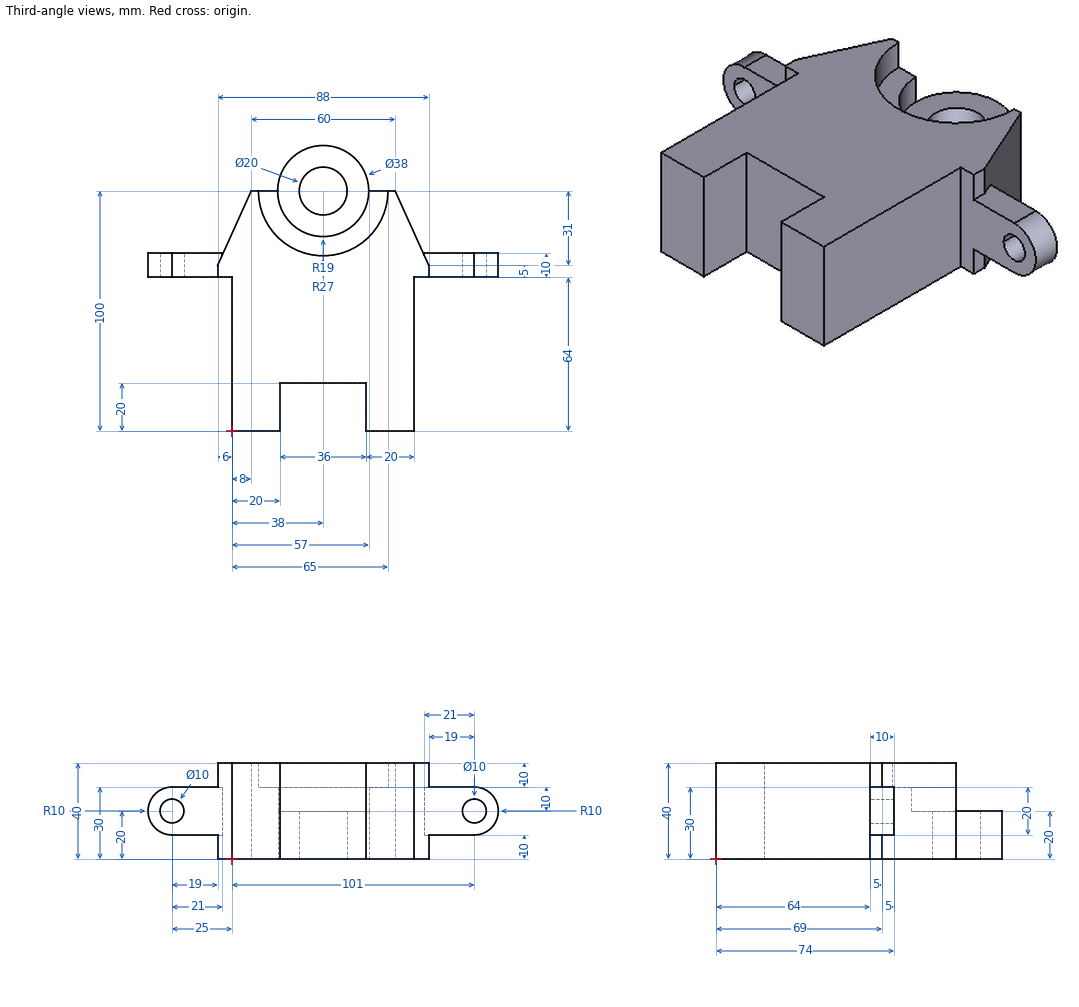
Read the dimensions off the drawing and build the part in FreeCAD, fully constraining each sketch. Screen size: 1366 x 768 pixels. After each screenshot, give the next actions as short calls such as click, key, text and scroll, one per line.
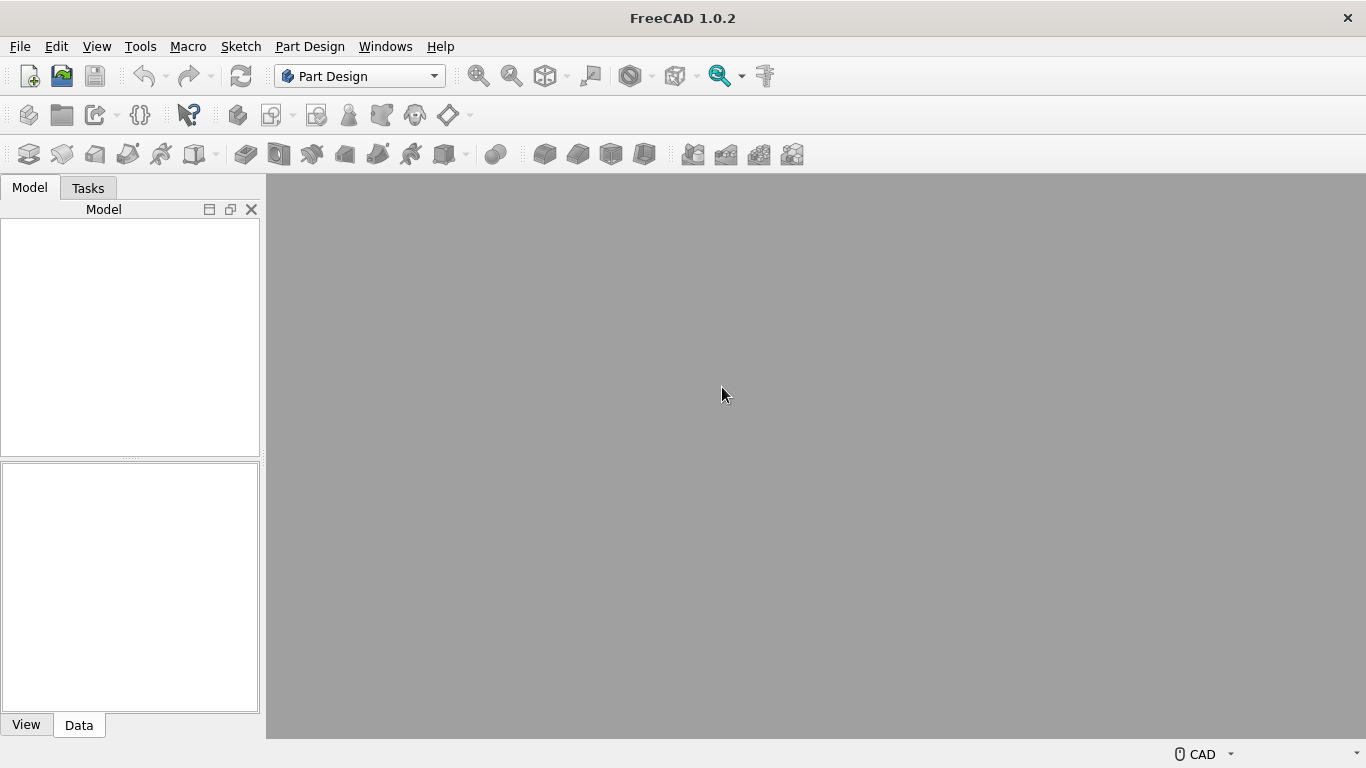
click(29, 76)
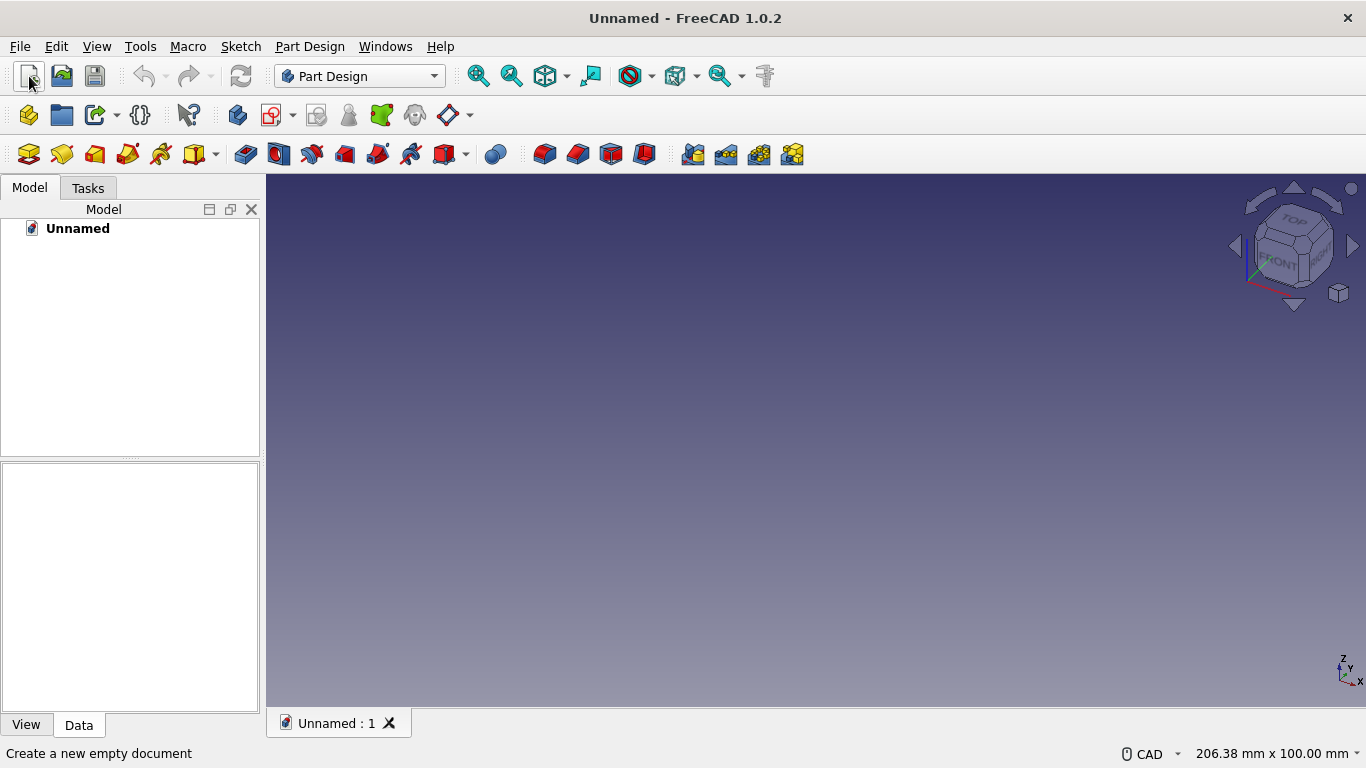
click(270, 116)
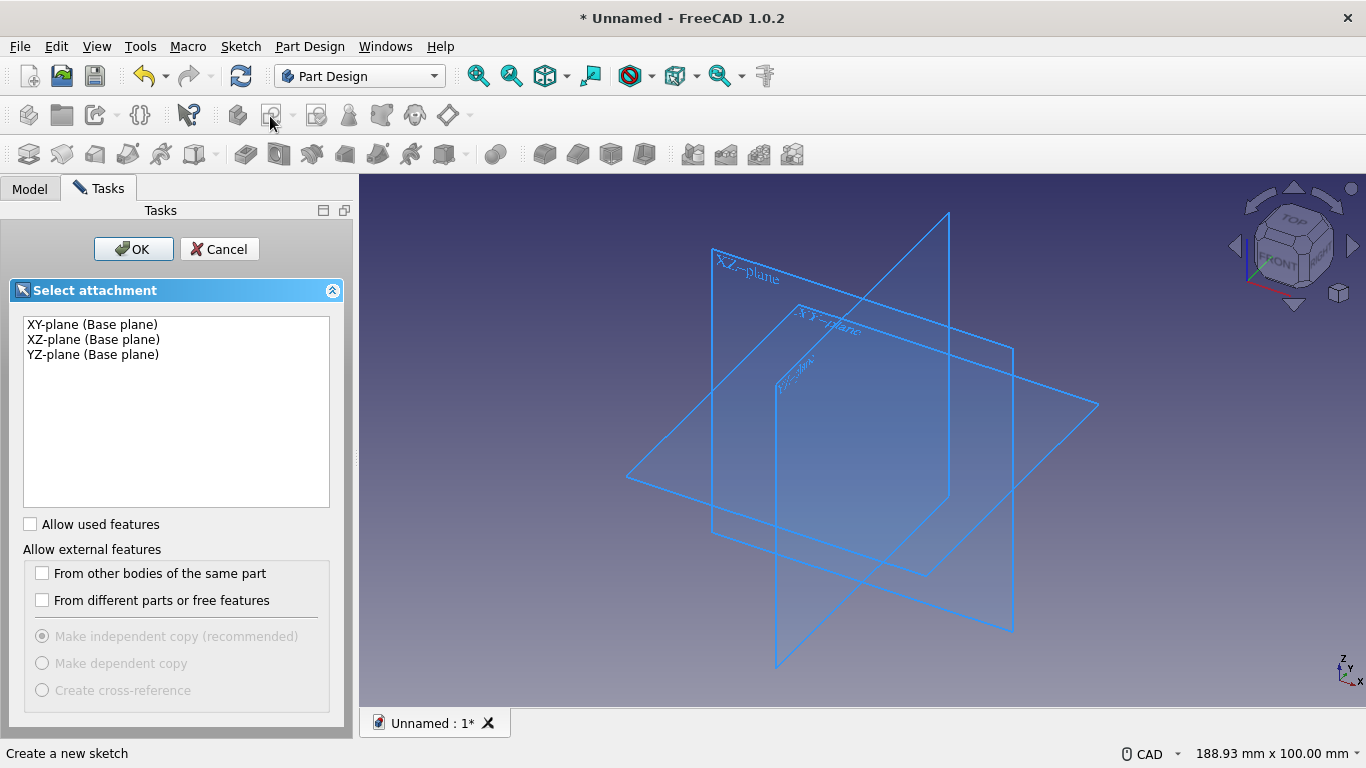
click(84, 324)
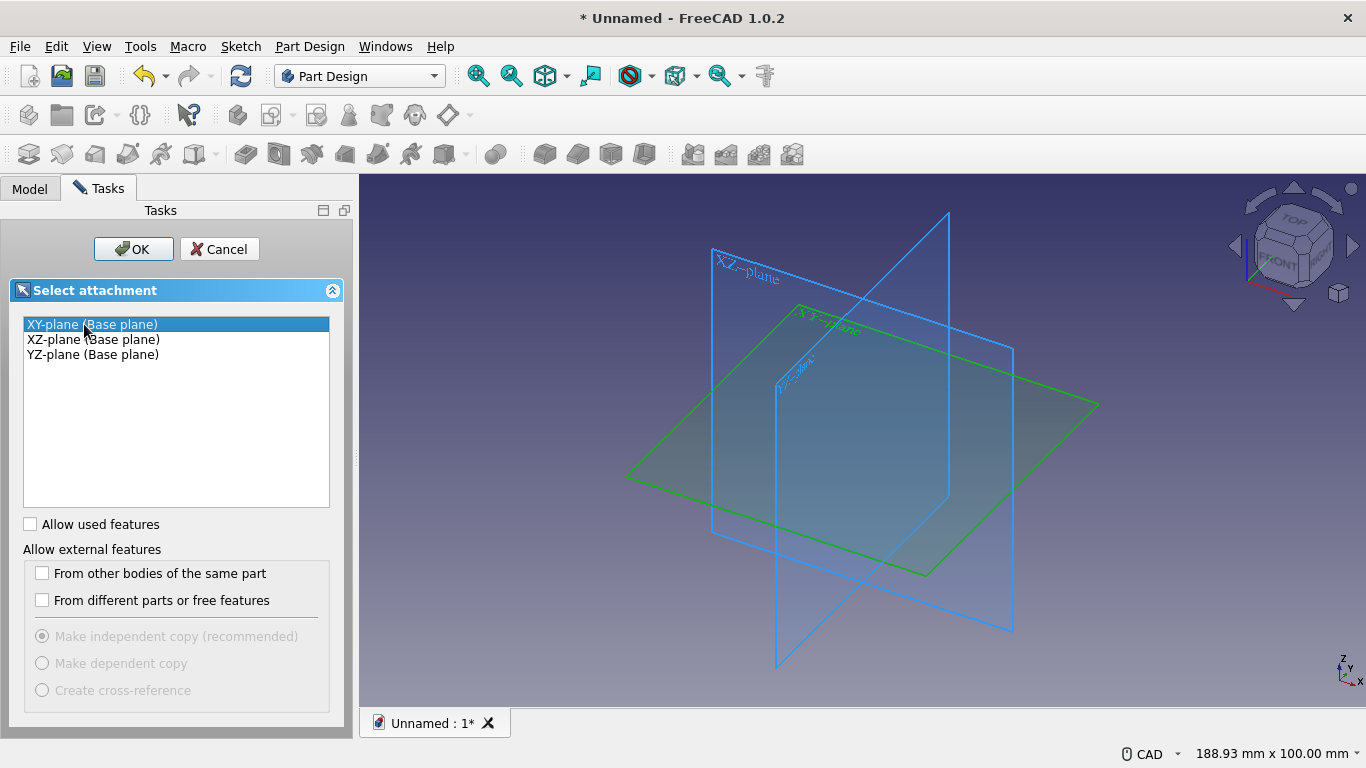
click(134, 249)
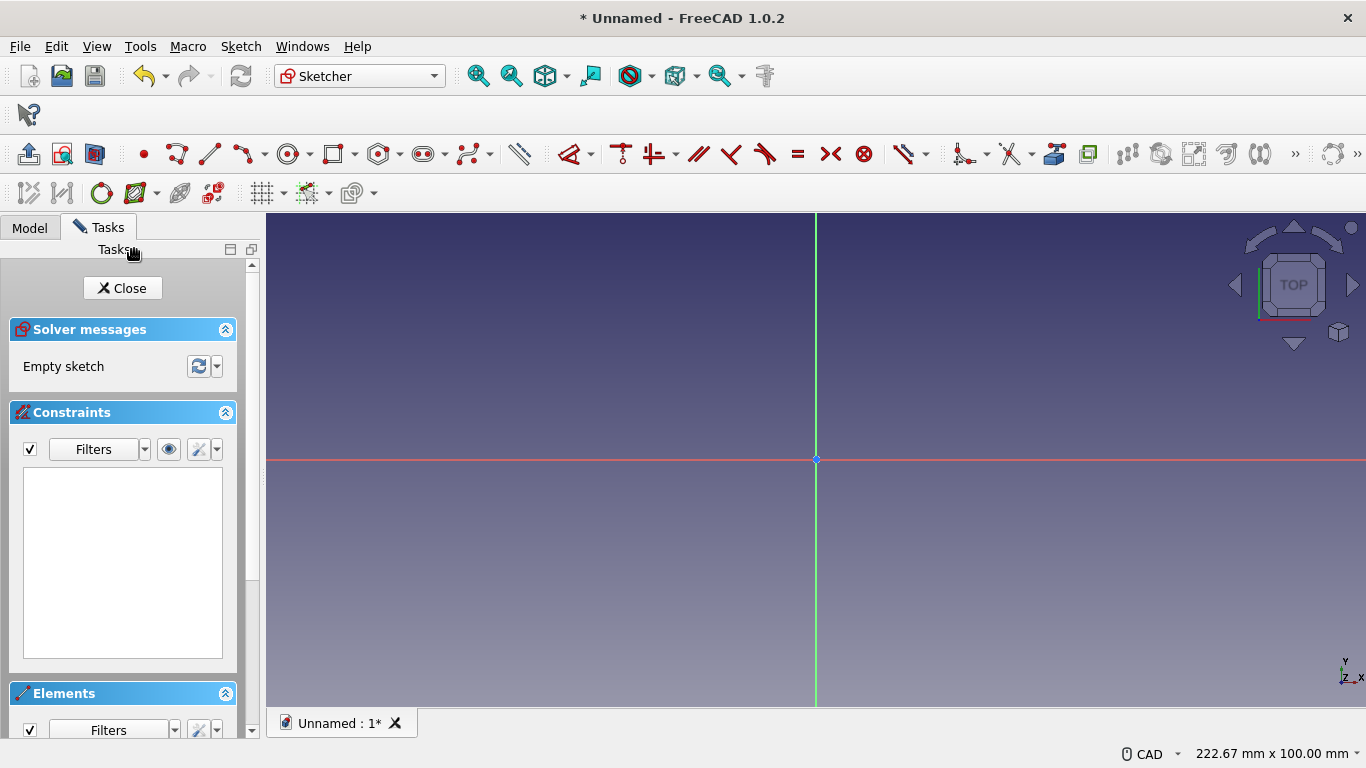
scroll(294, 679, down, 2)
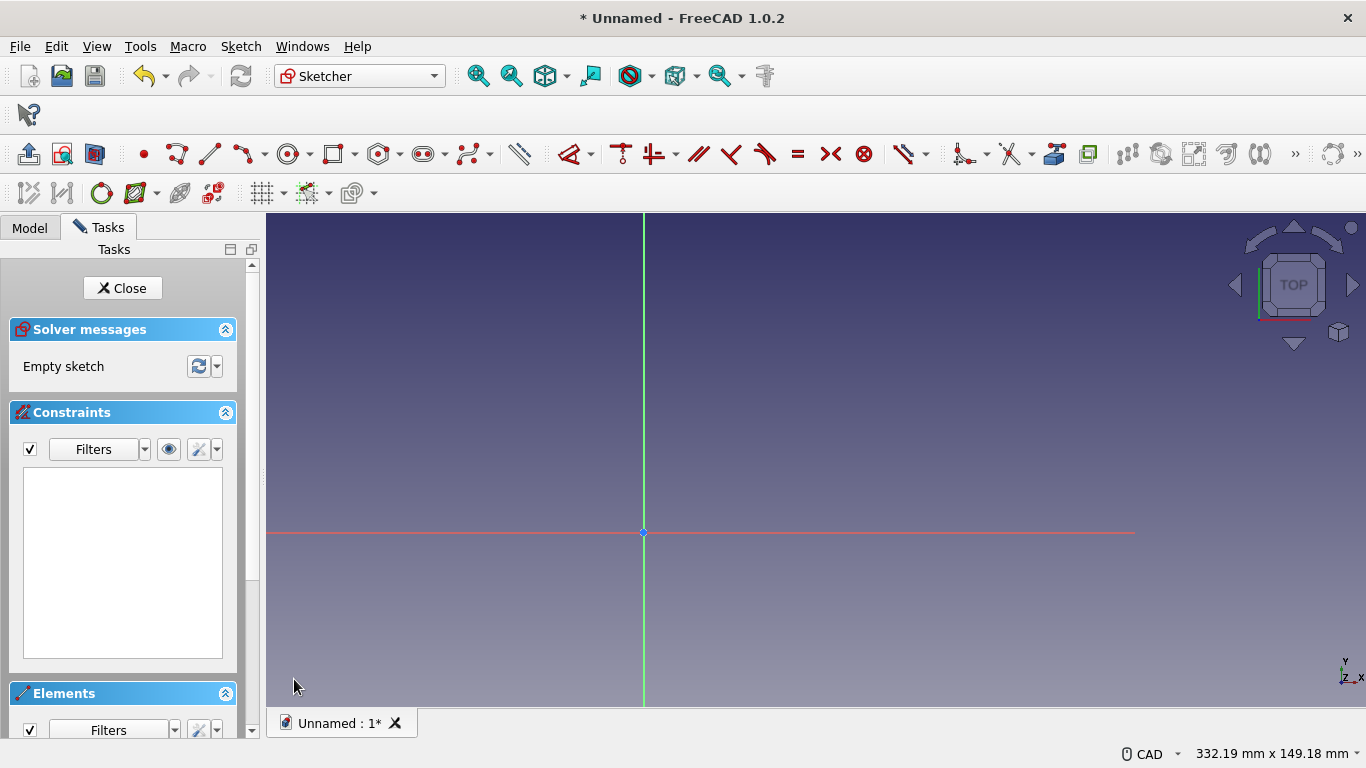
scroll(815, 359, up, 2)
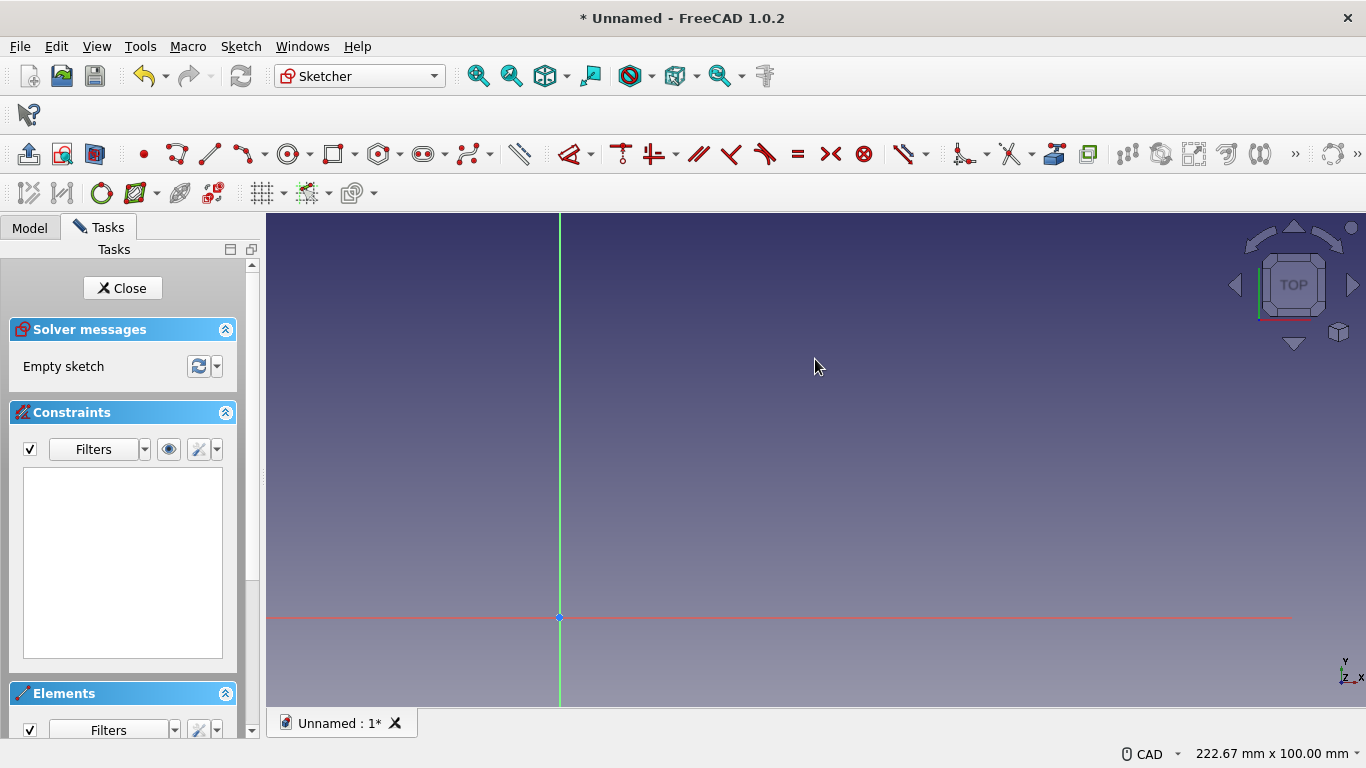
click(177, 154)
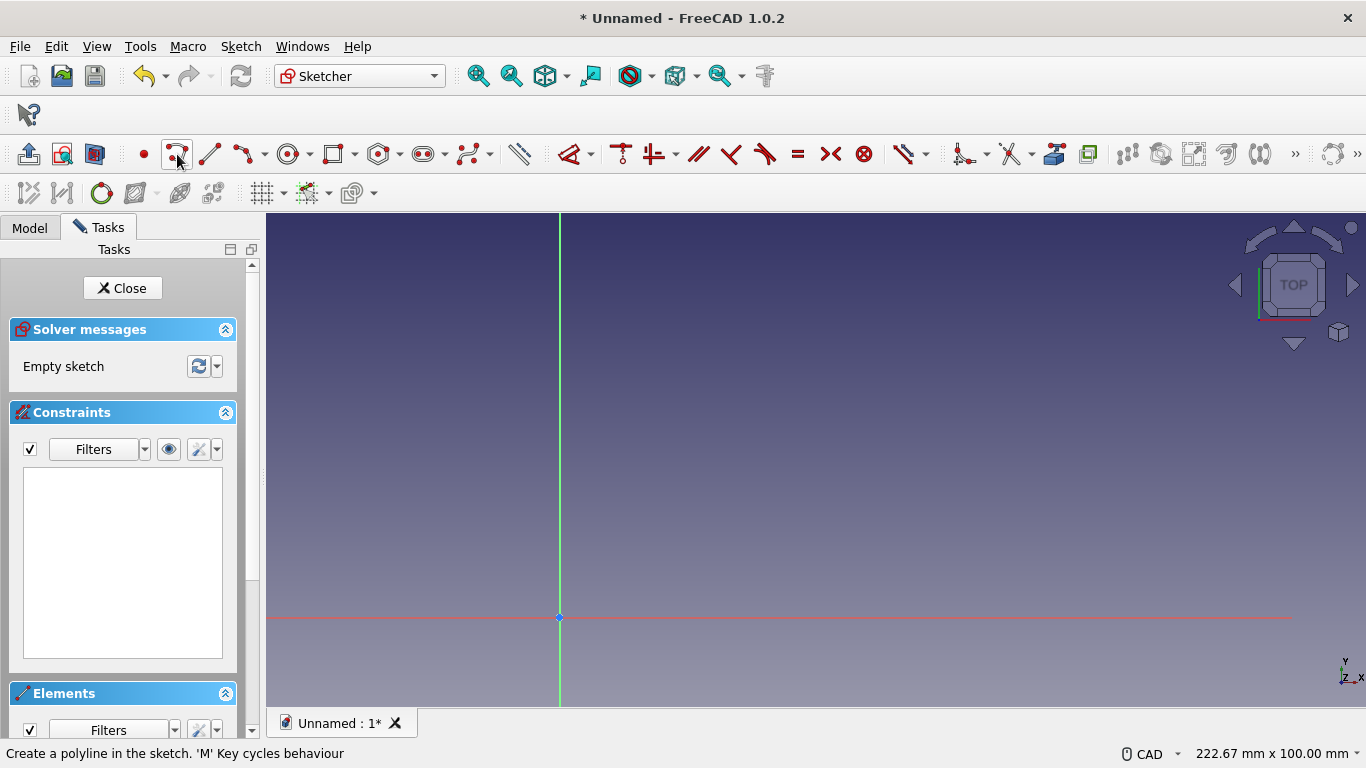
click(560, 618)
click(658, 609)
click(658, 519)
click(836, 519)
click(836, 618)
click(935, 609)
click(935, 302)
click(569, 302)
click(560, 618)
key(Escape)
key(Escape)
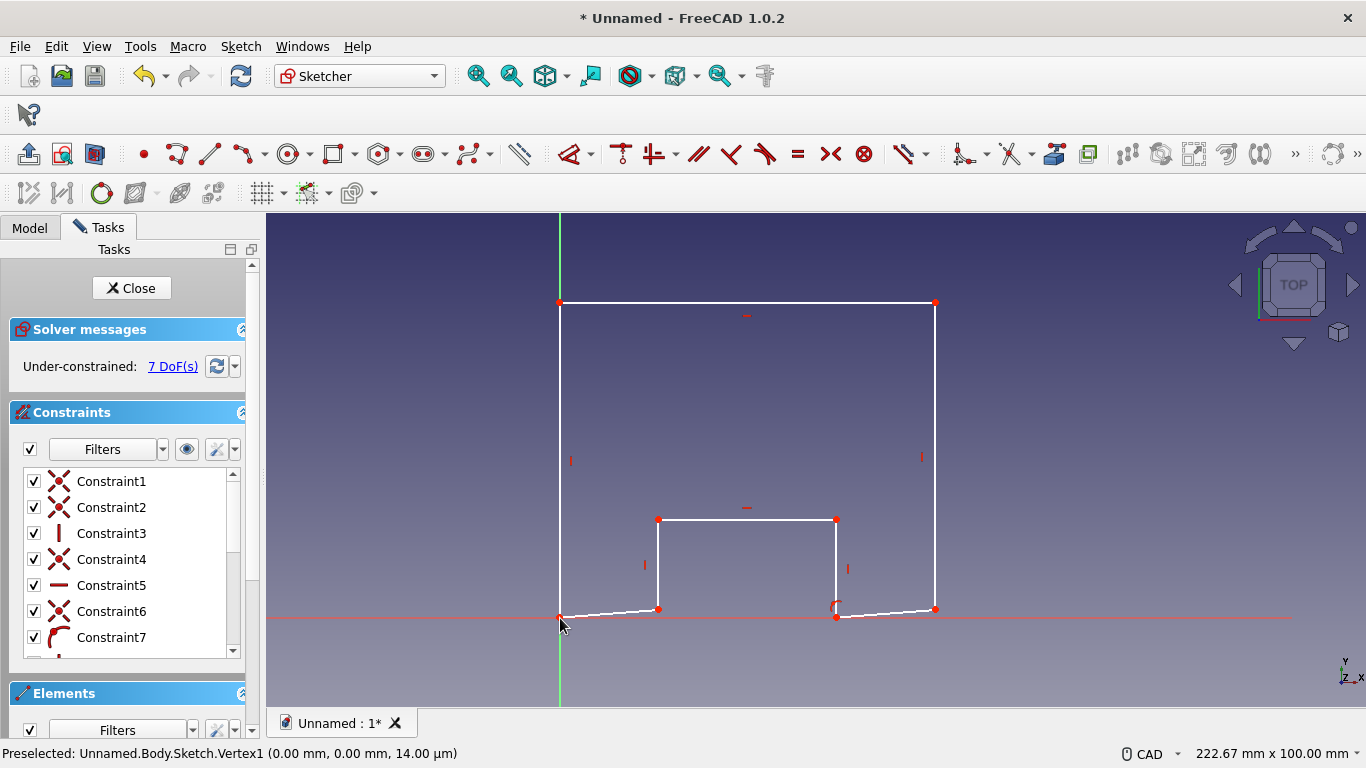
click(589, 615)